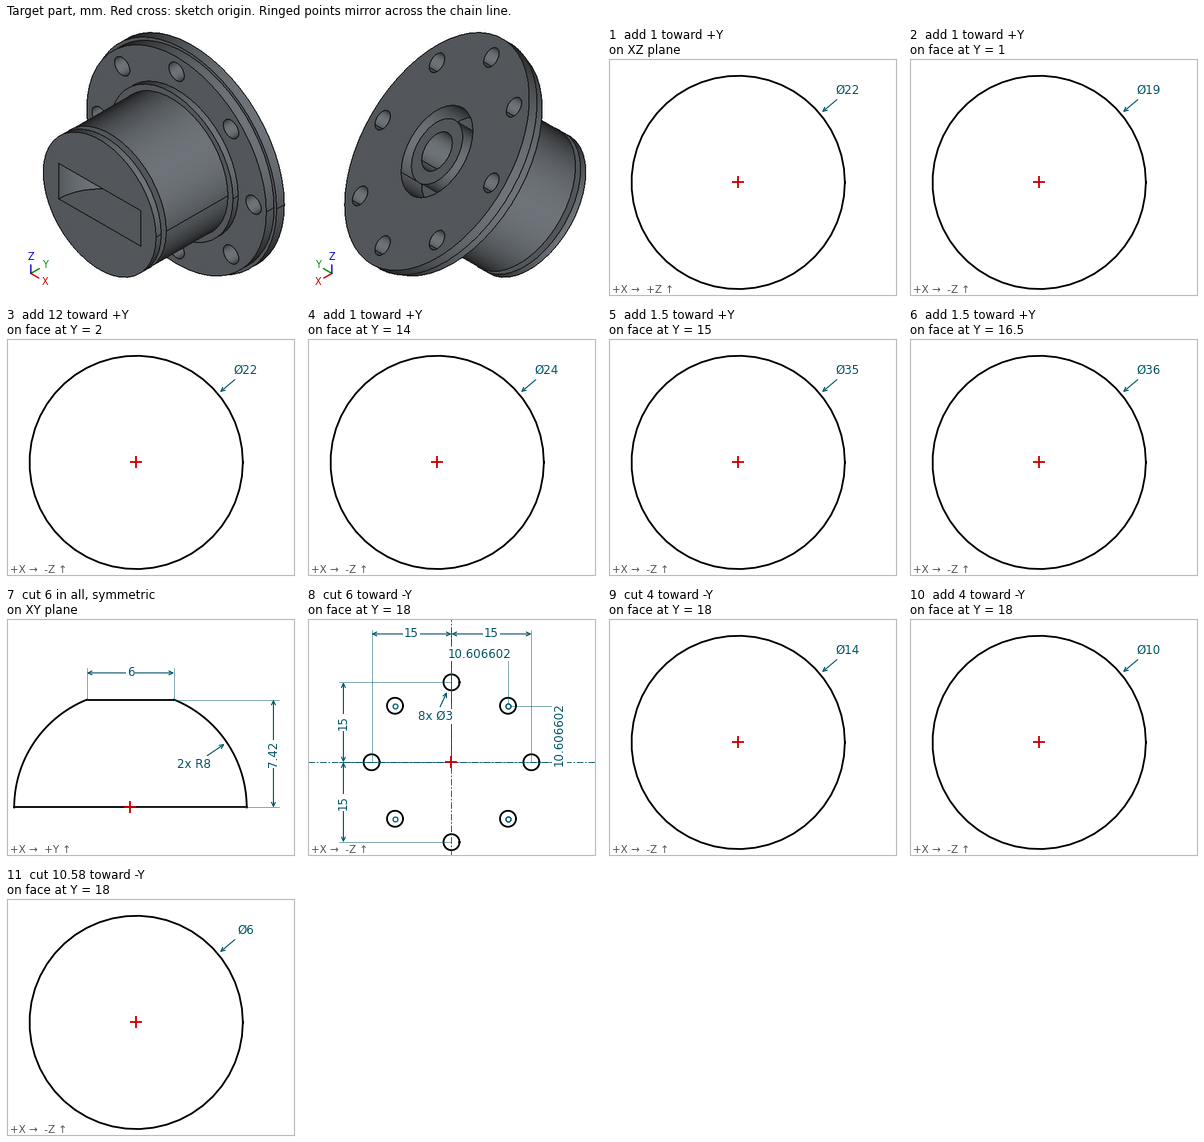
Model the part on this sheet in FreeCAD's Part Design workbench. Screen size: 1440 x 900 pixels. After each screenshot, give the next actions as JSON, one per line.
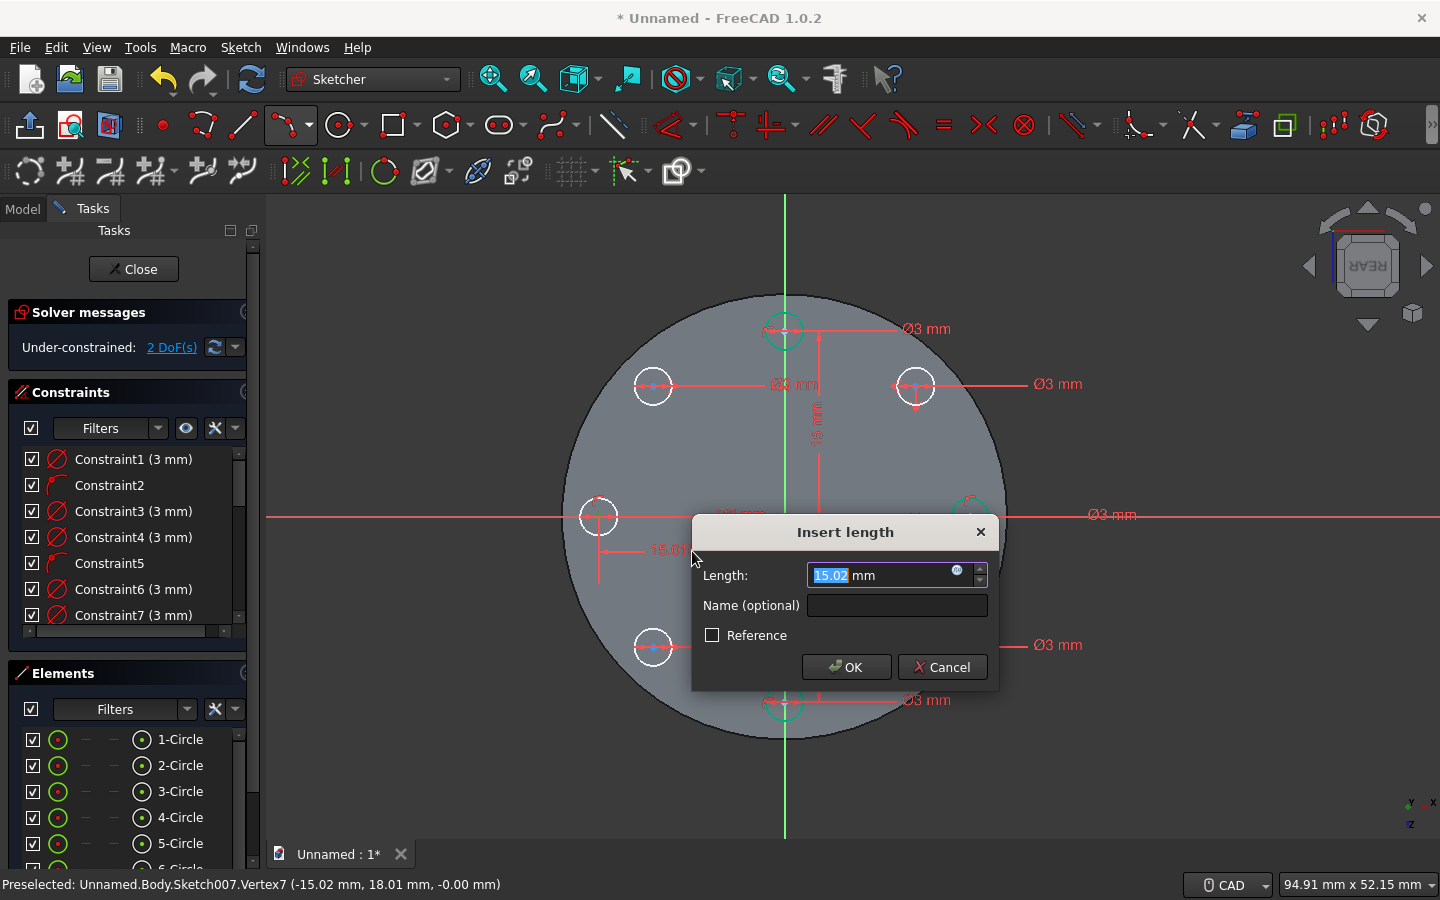
{"action": "type", "text": "15"}
{"action": "key", "text": "Return"}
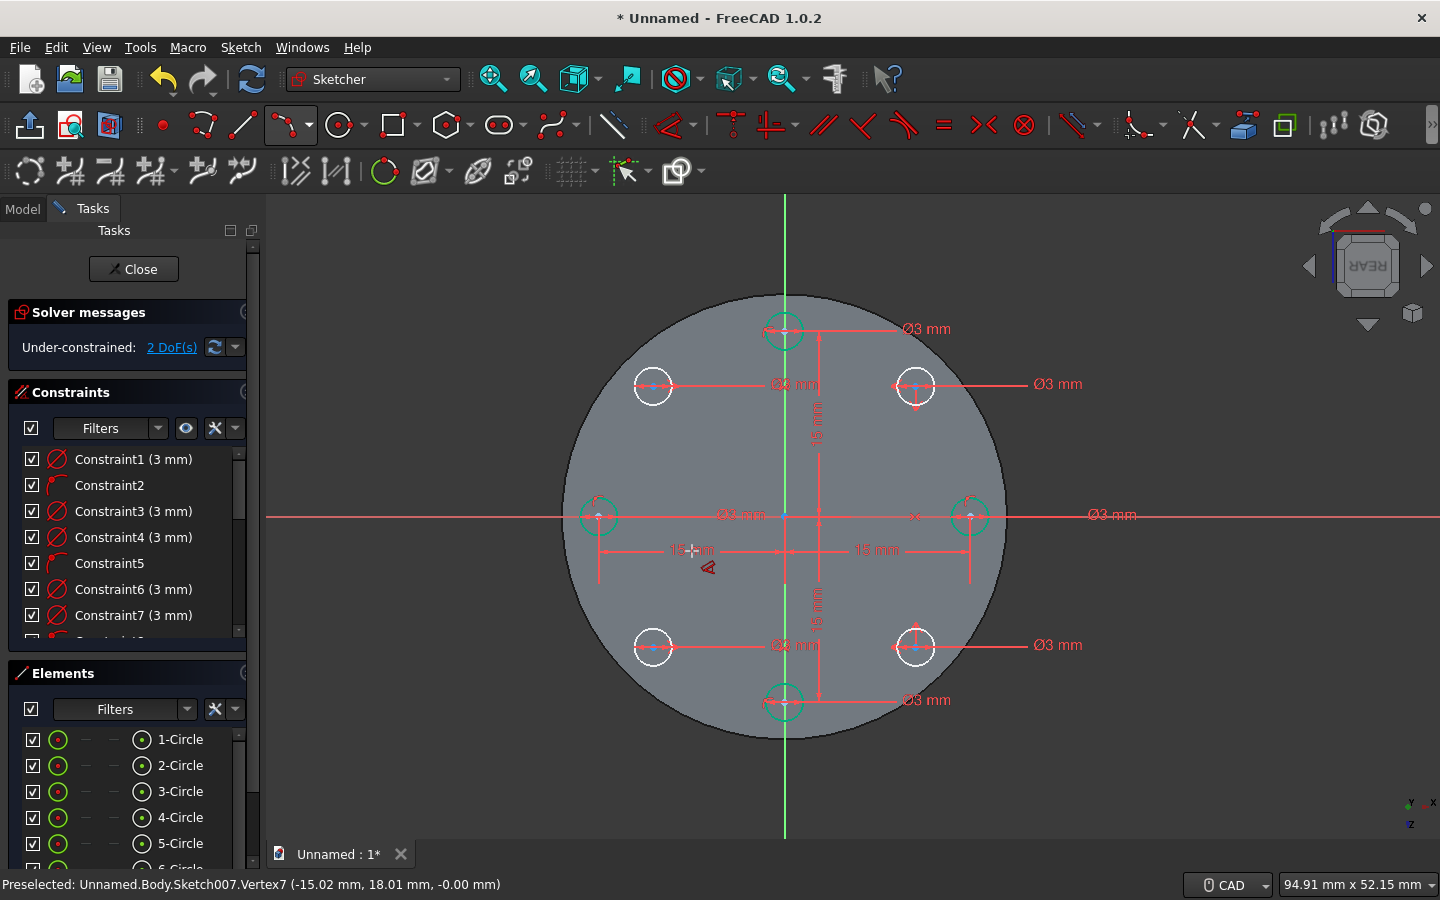
{"action": "left_click", "coordinate": [916, 386]}
{"action": "left_click", "coordinate": [850, 352]}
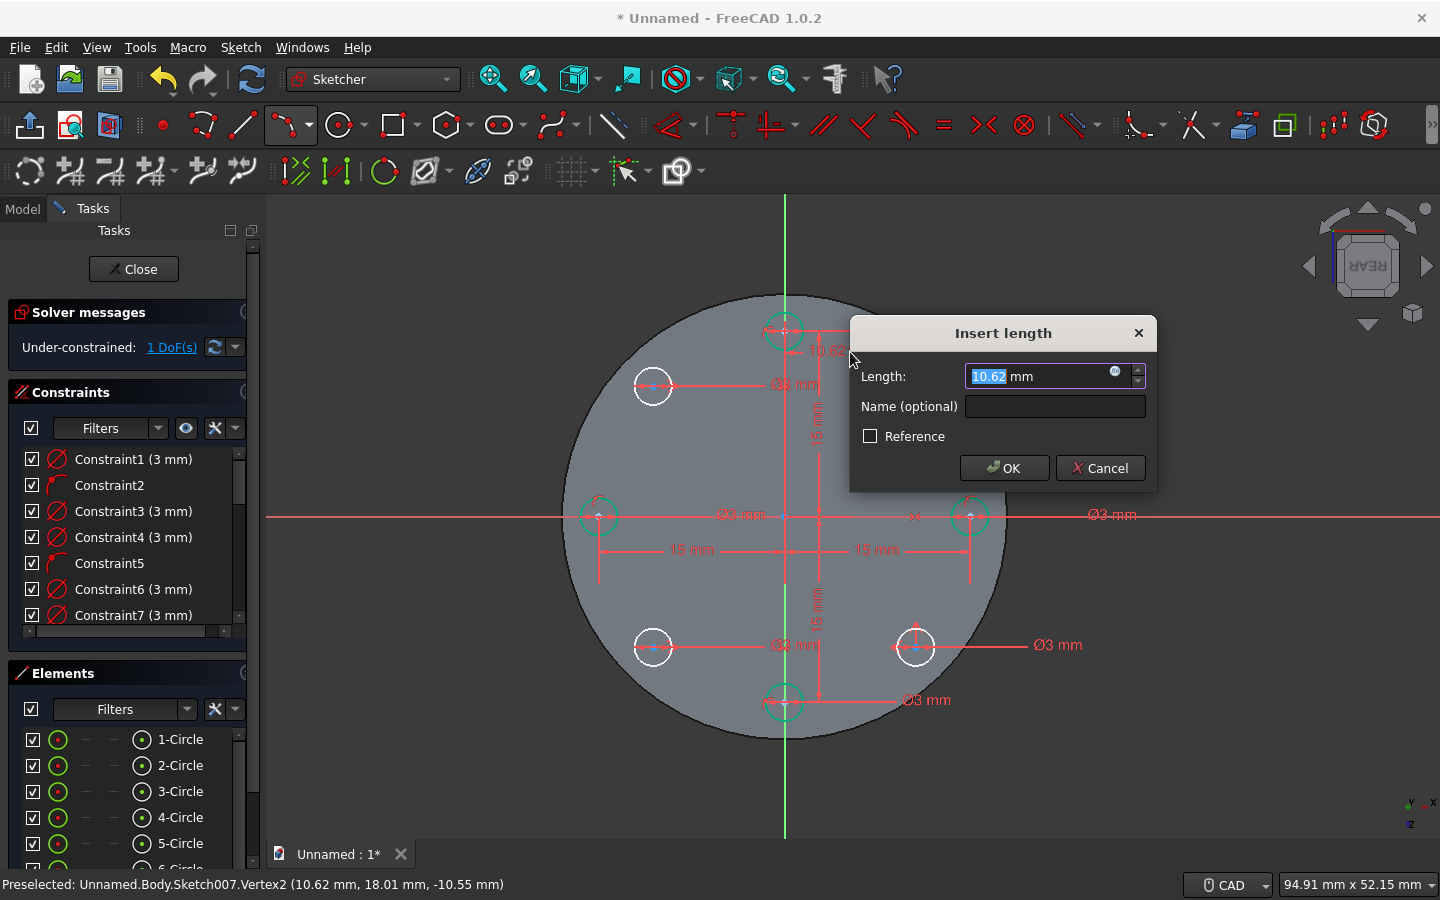
{"action": "type", "text": "10.606602"}
{"action": "key", "text": "Return"}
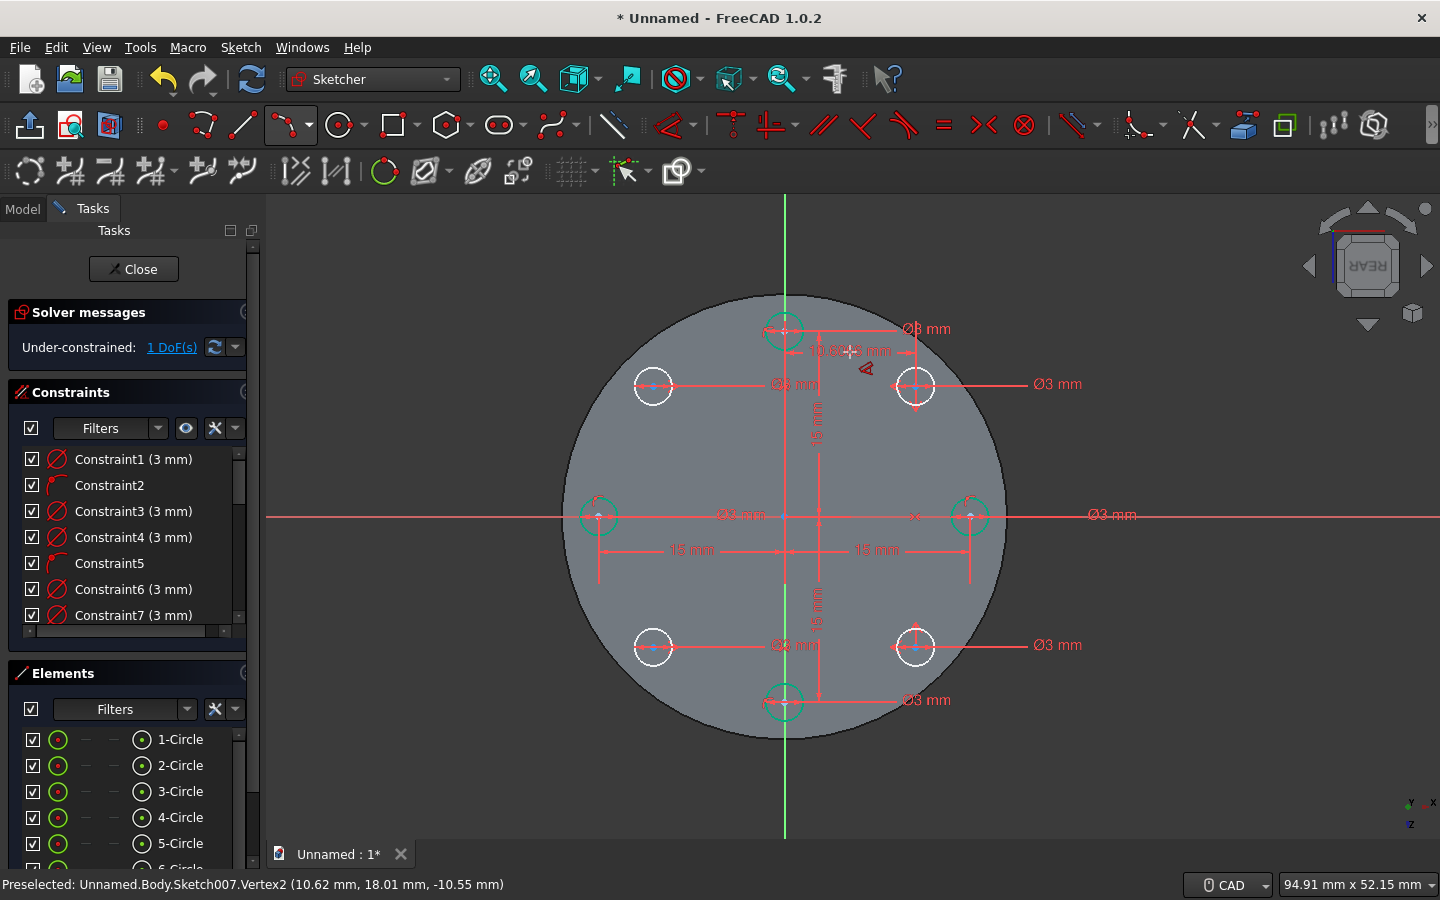
{"action": "left_click", "coordinate": [916, 386]}
{"action": "left_click", "coordinate": [950, 452]}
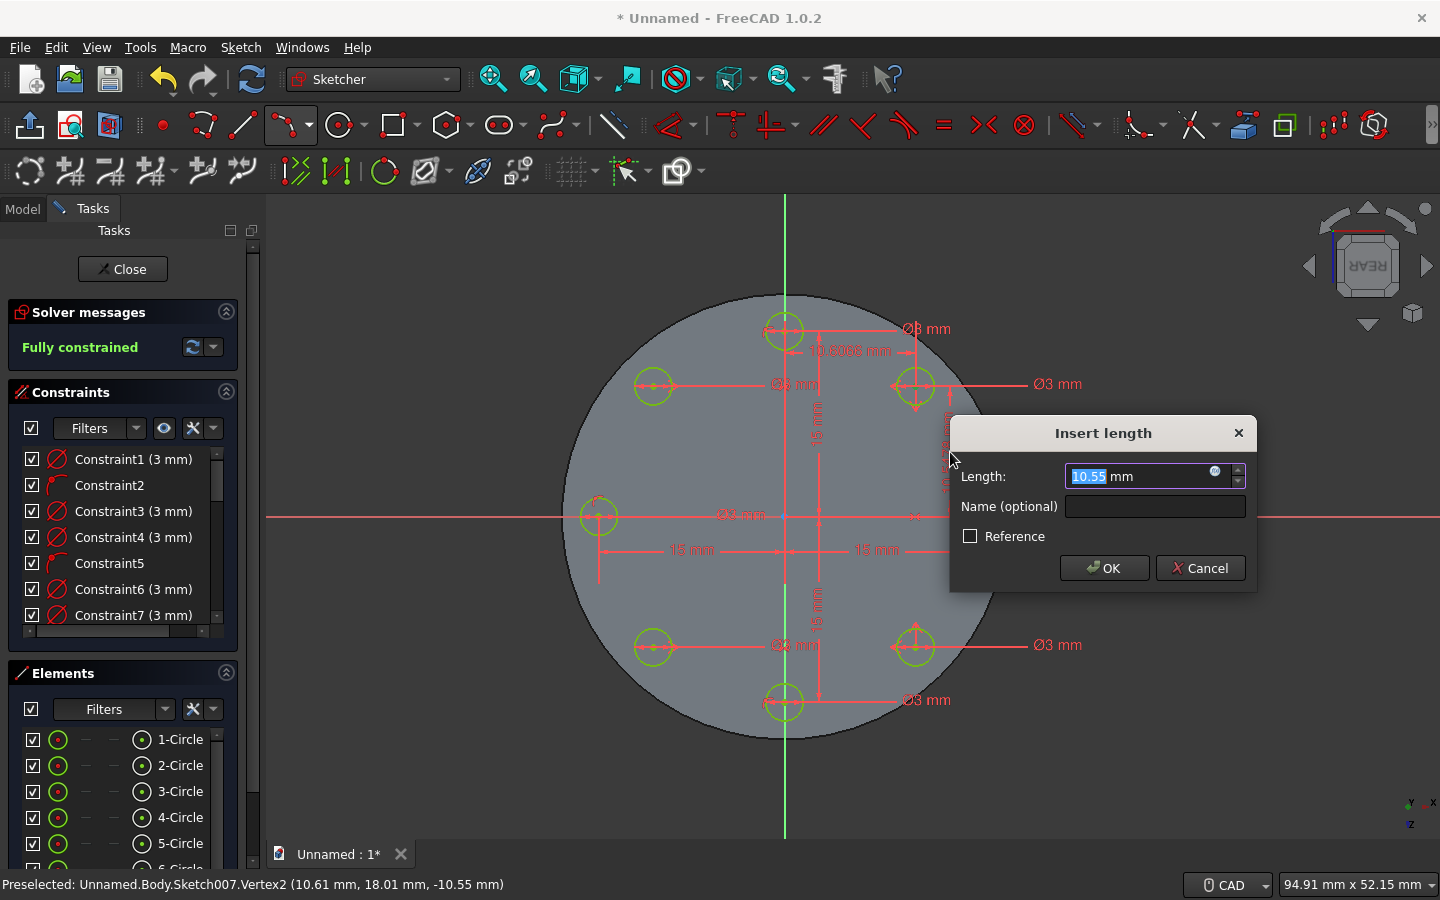
{"action": "type", "text": "10.606602"}
{"action": "key", "text": "Return"}
{"action": "key", "text": "Escape"}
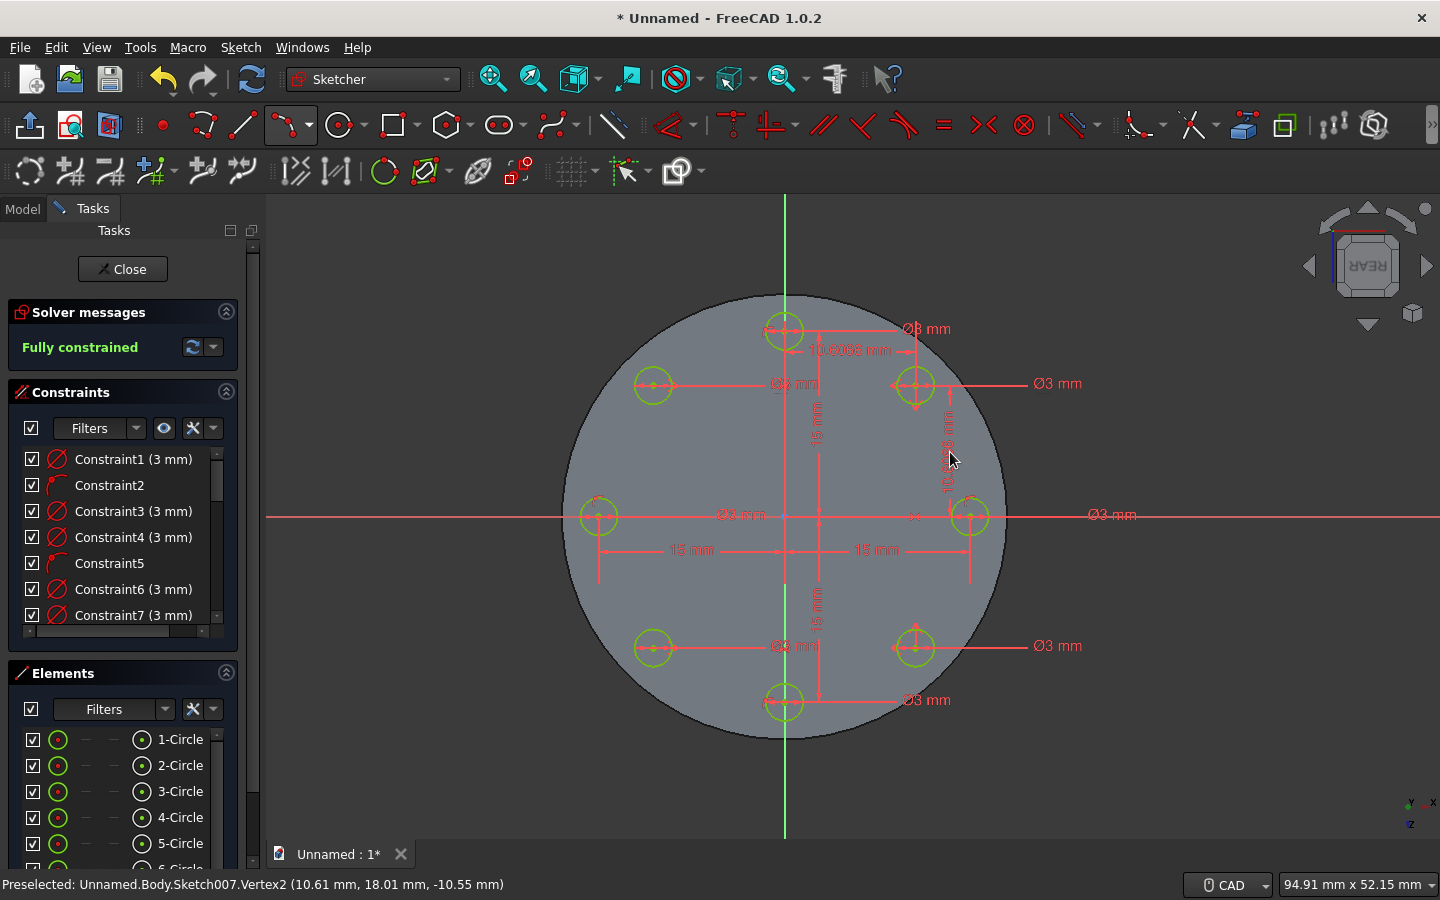
{"action": "left_click", "coordinate": [123, 269]}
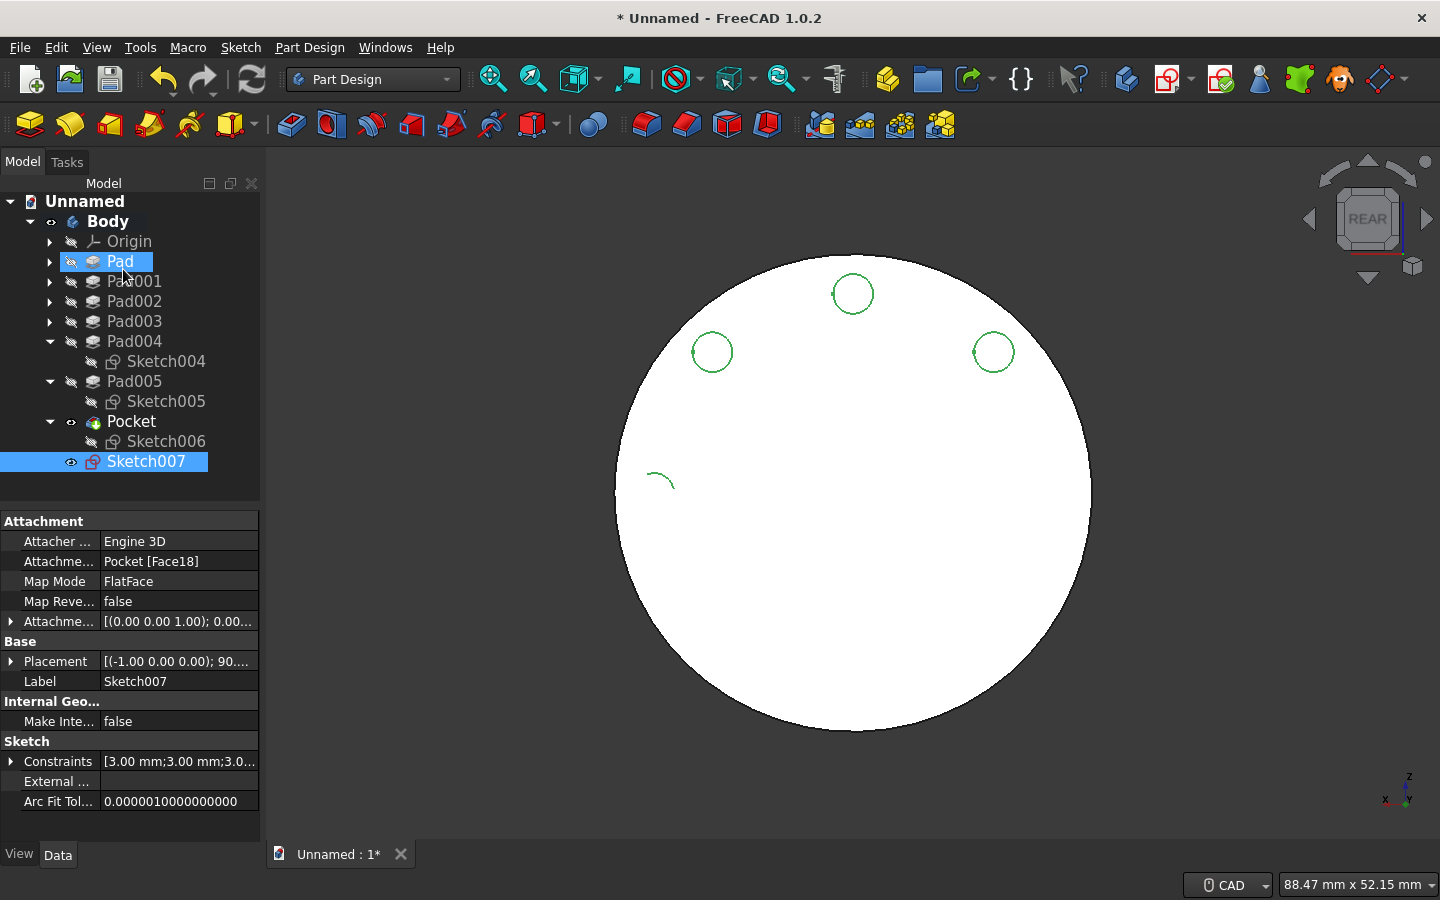
{"action": "left_click", "coordinate": [292, 124]}